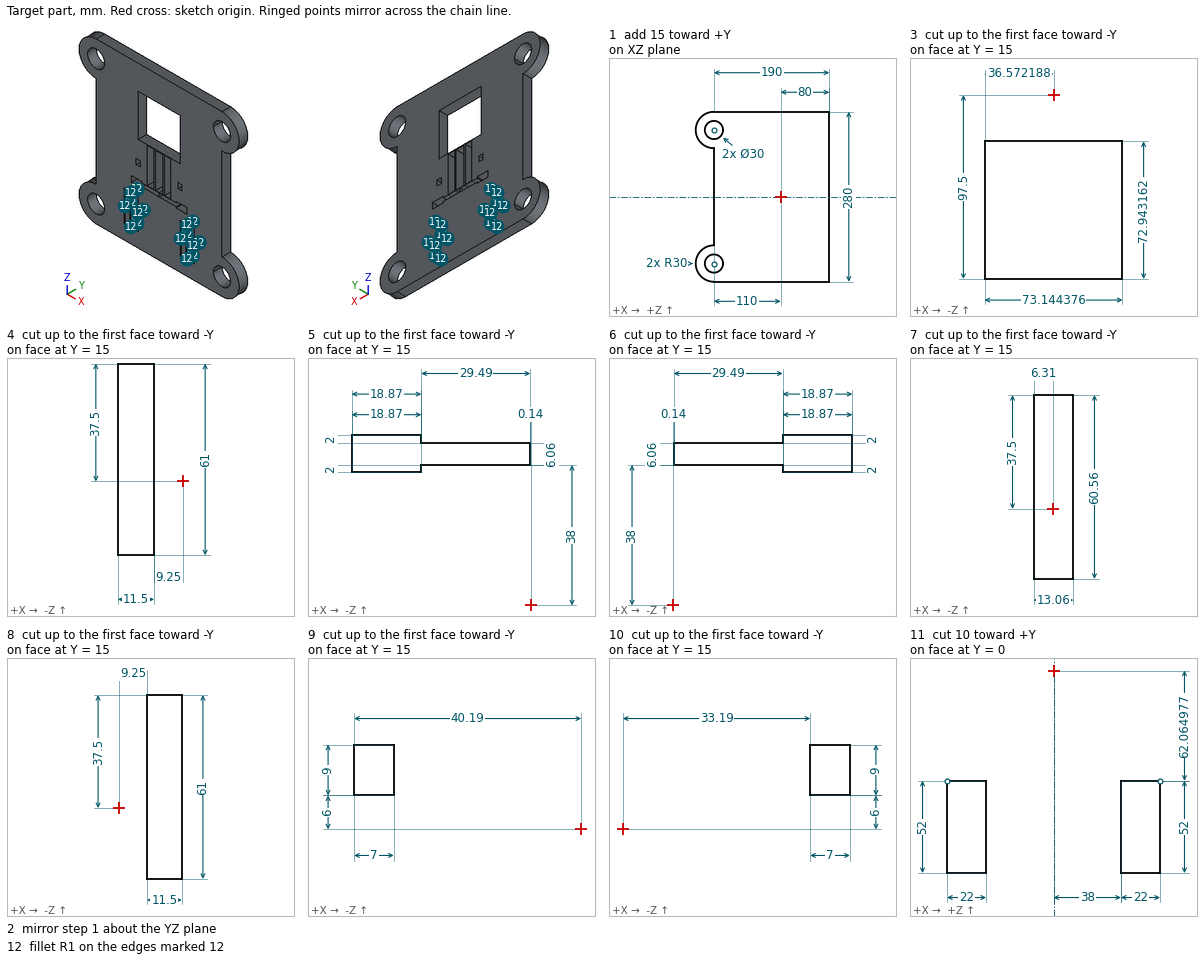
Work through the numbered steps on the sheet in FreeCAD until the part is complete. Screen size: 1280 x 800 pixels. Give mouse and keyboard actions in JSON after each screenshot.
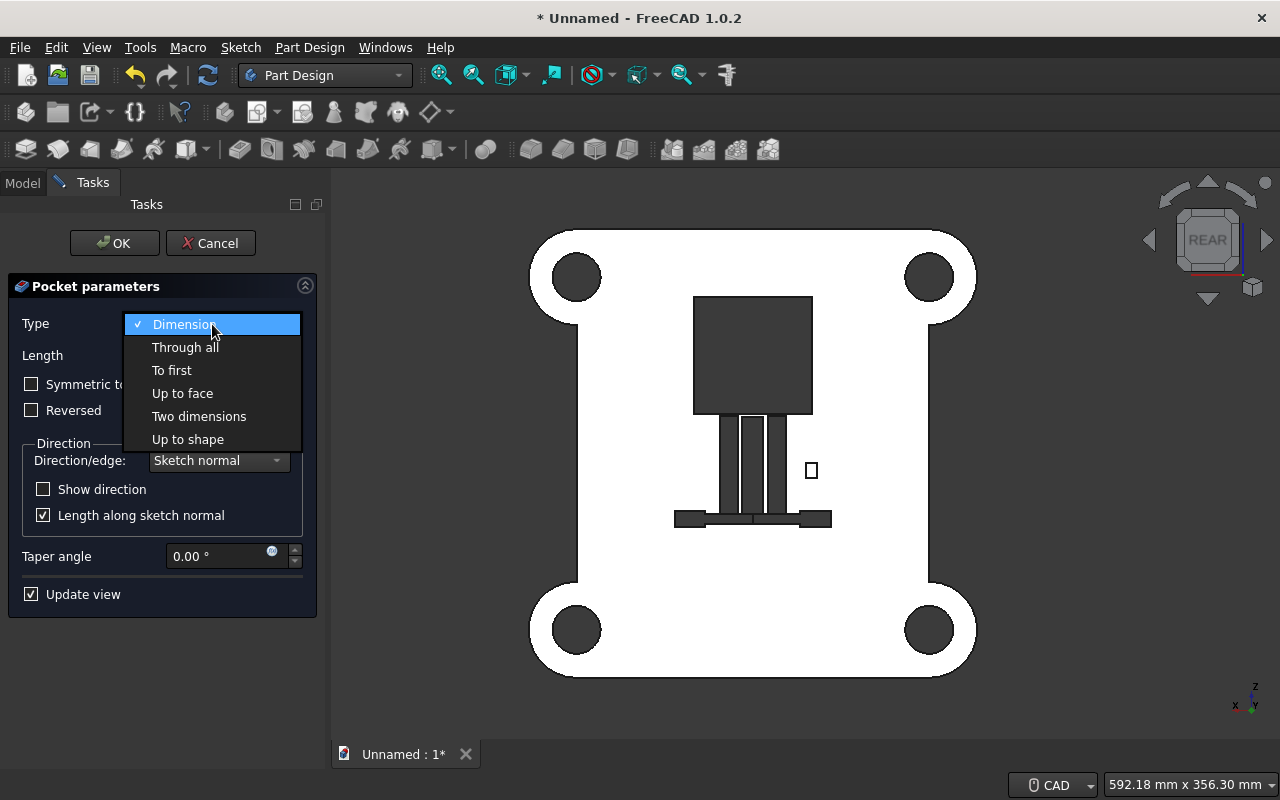
{"action": "left_click", "coordinate": [212, 370]}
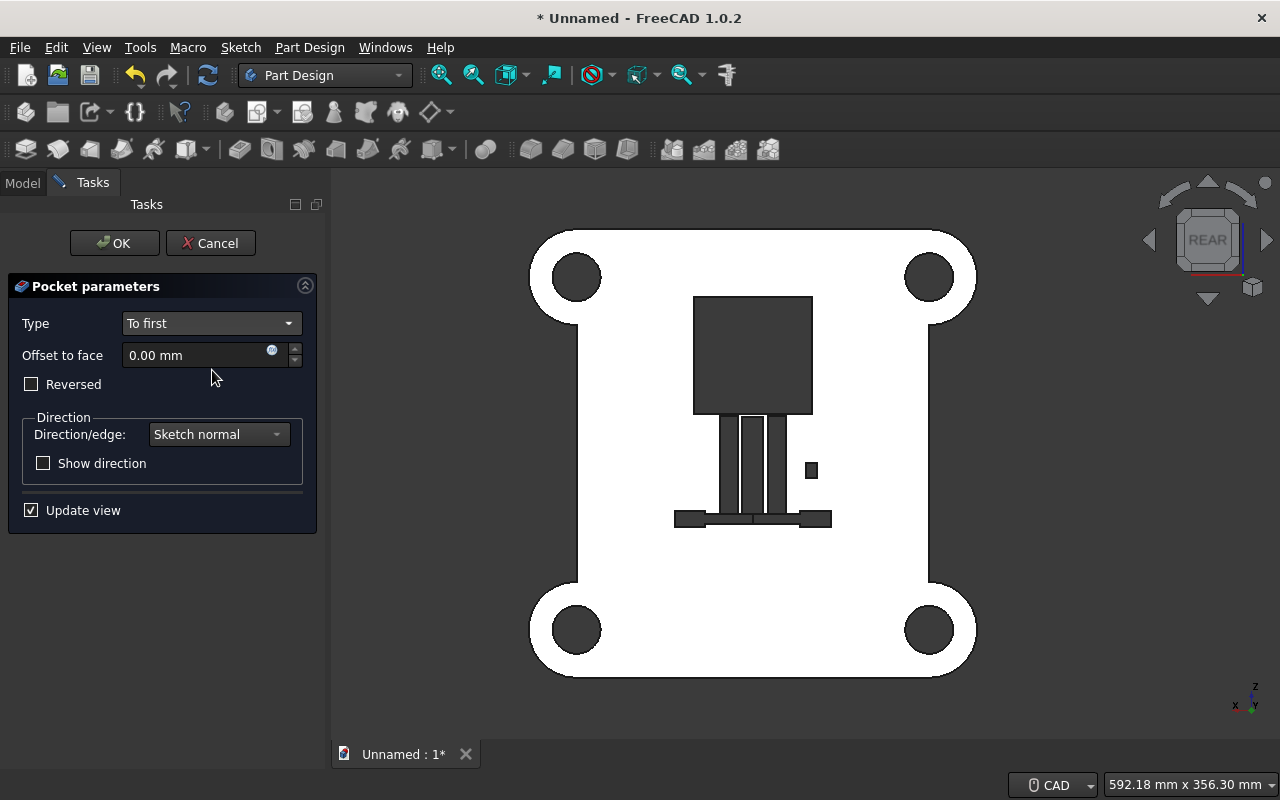
{"action": "left_click", "coordinate": [115, 243]}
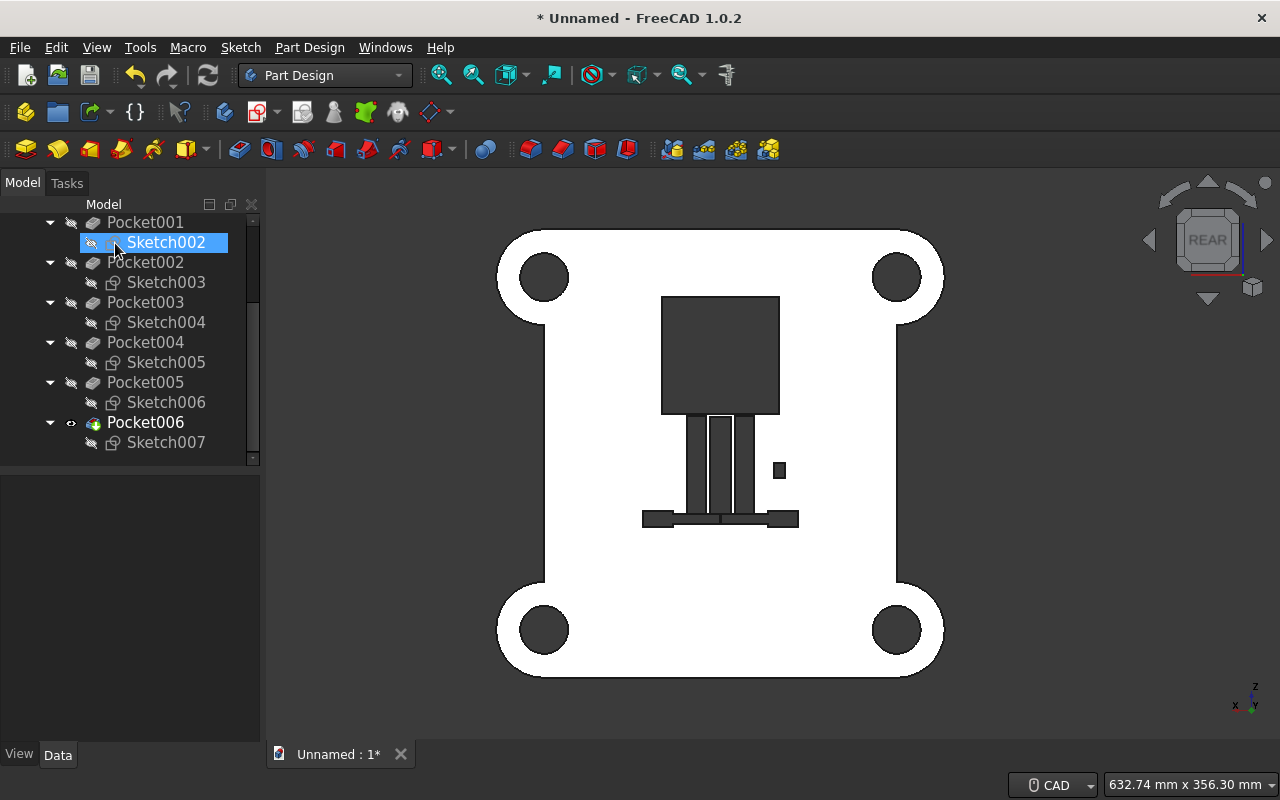
{"action": "left_click", "coordinate": [720, 581]}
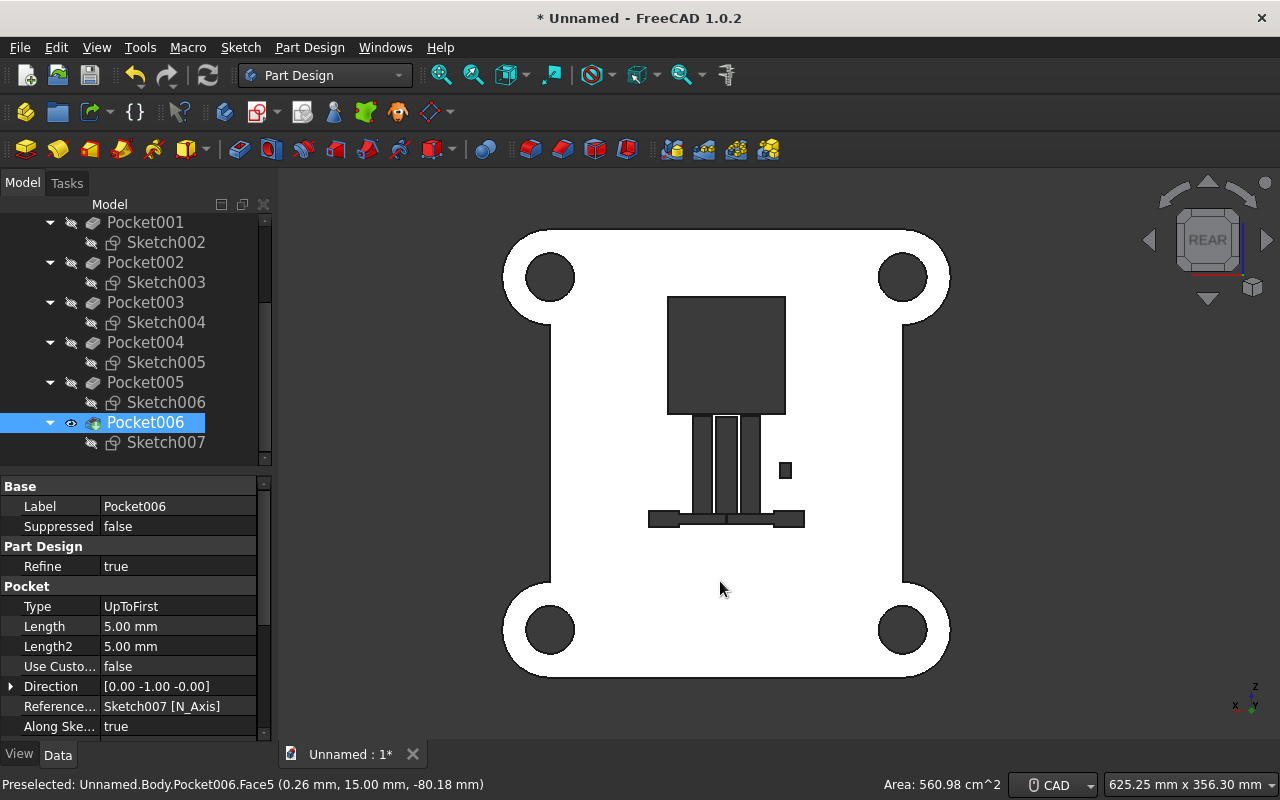
{"action": "left_click", "coordinate": [258, 112]}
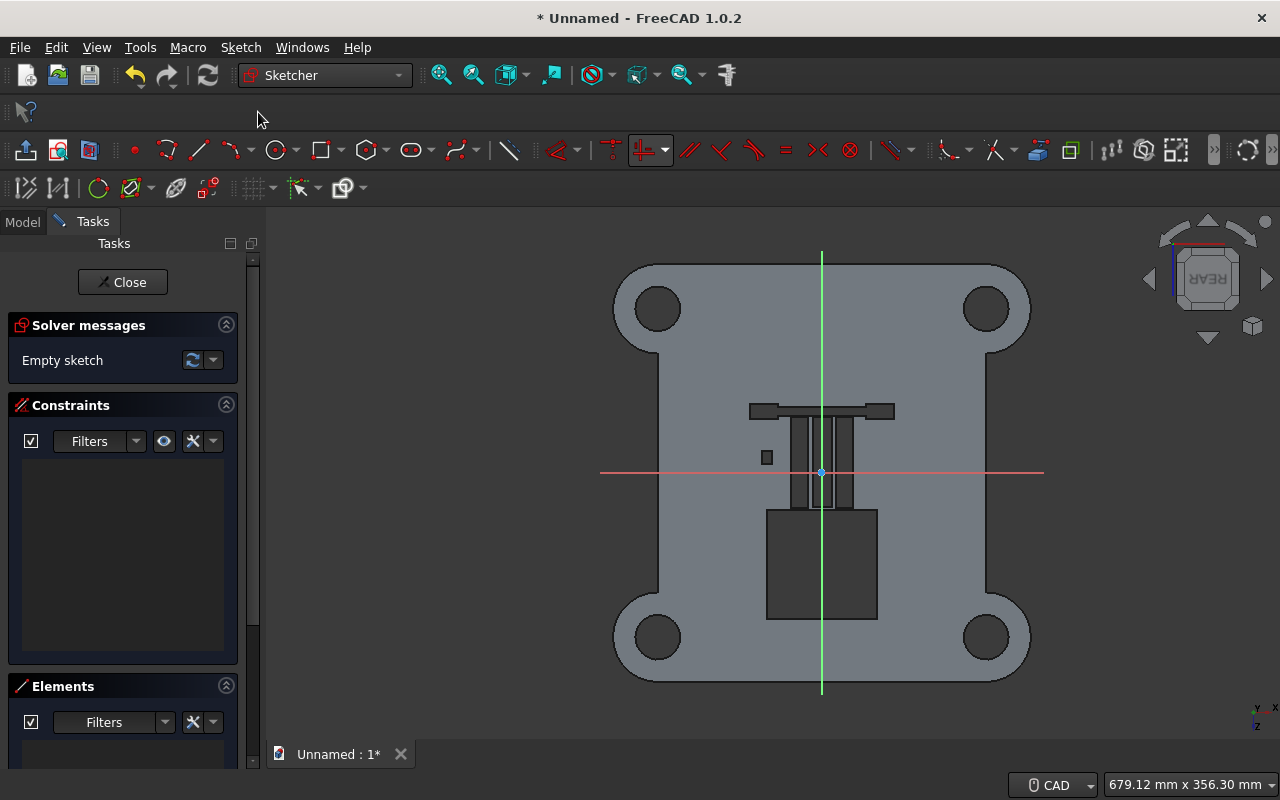
{"action": "scroll", "coordinate": [886, 457], "scroll_direction": "up", "scroll_amount": 15}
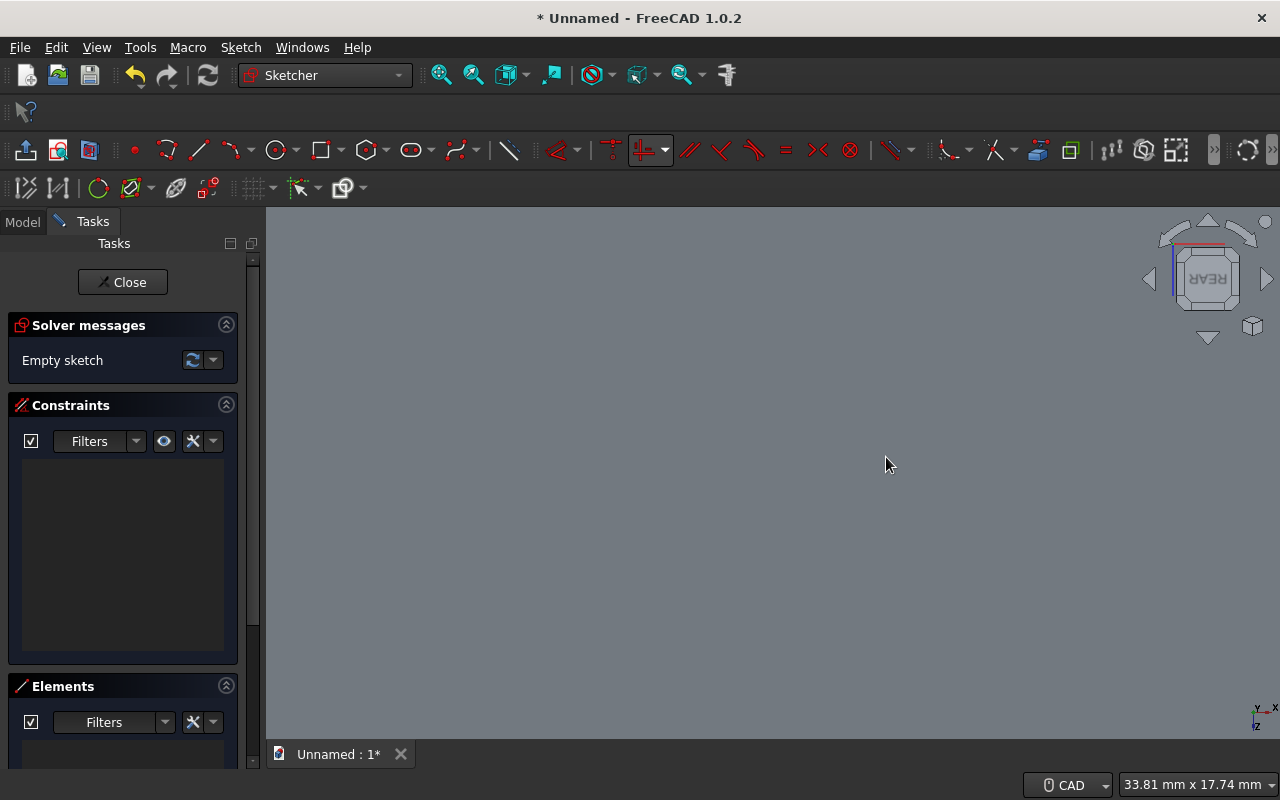
{"action": "key", "text": "g r"}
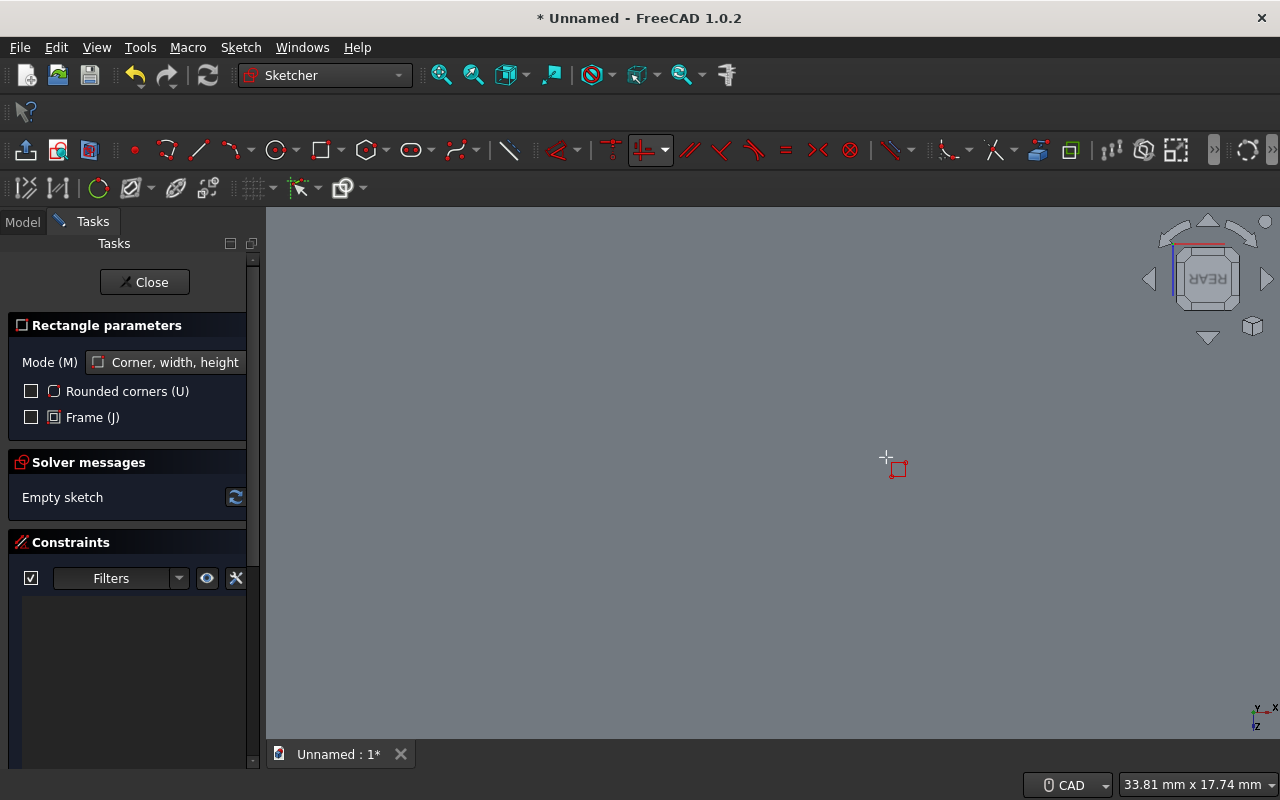
{"action": "left_click", "coordinate": [584, 320]}
{"action": "mouse_move", "coordinate": [794, 589]}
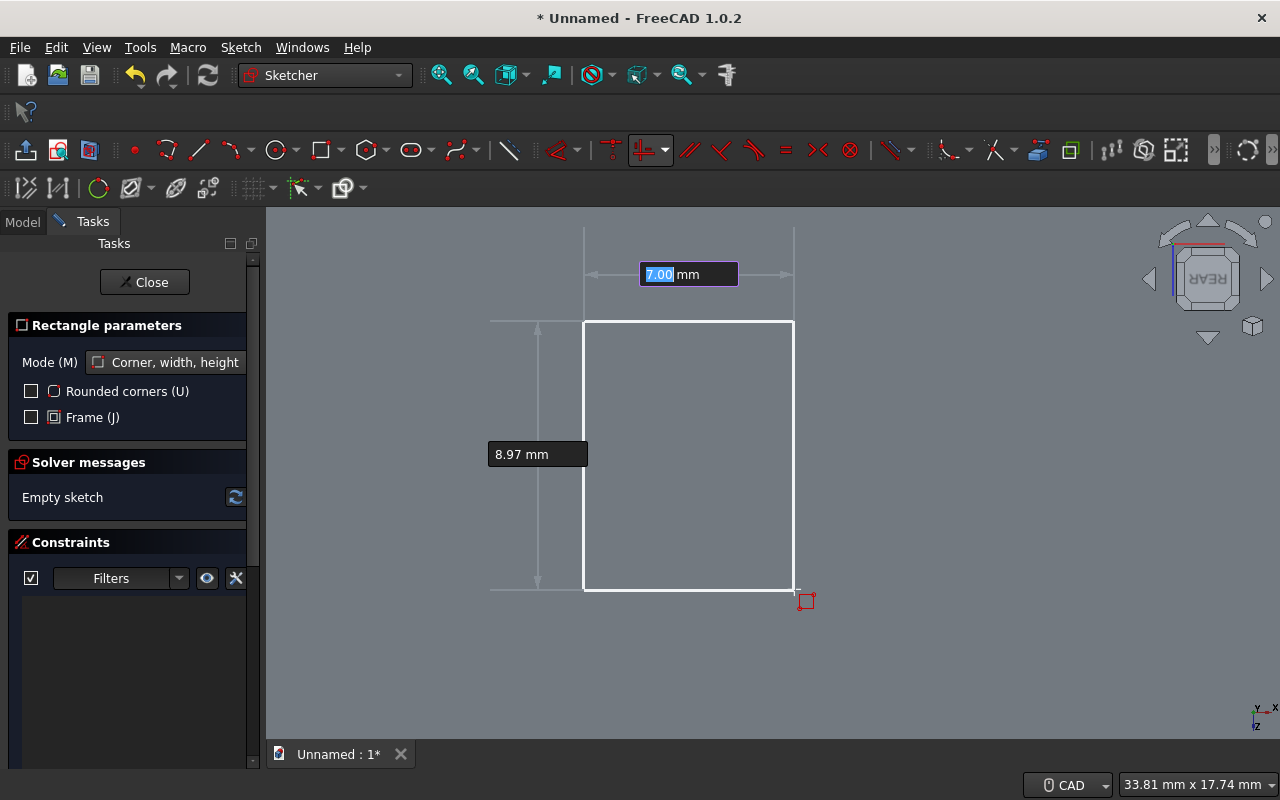
{"action": "type", "text": "7"}
{"action": "key", "text": "Tab"}
{"action": "type", "text": "9"}
{"action": "key", "text": "Return"}
{"action": "key", "text": "Escape"}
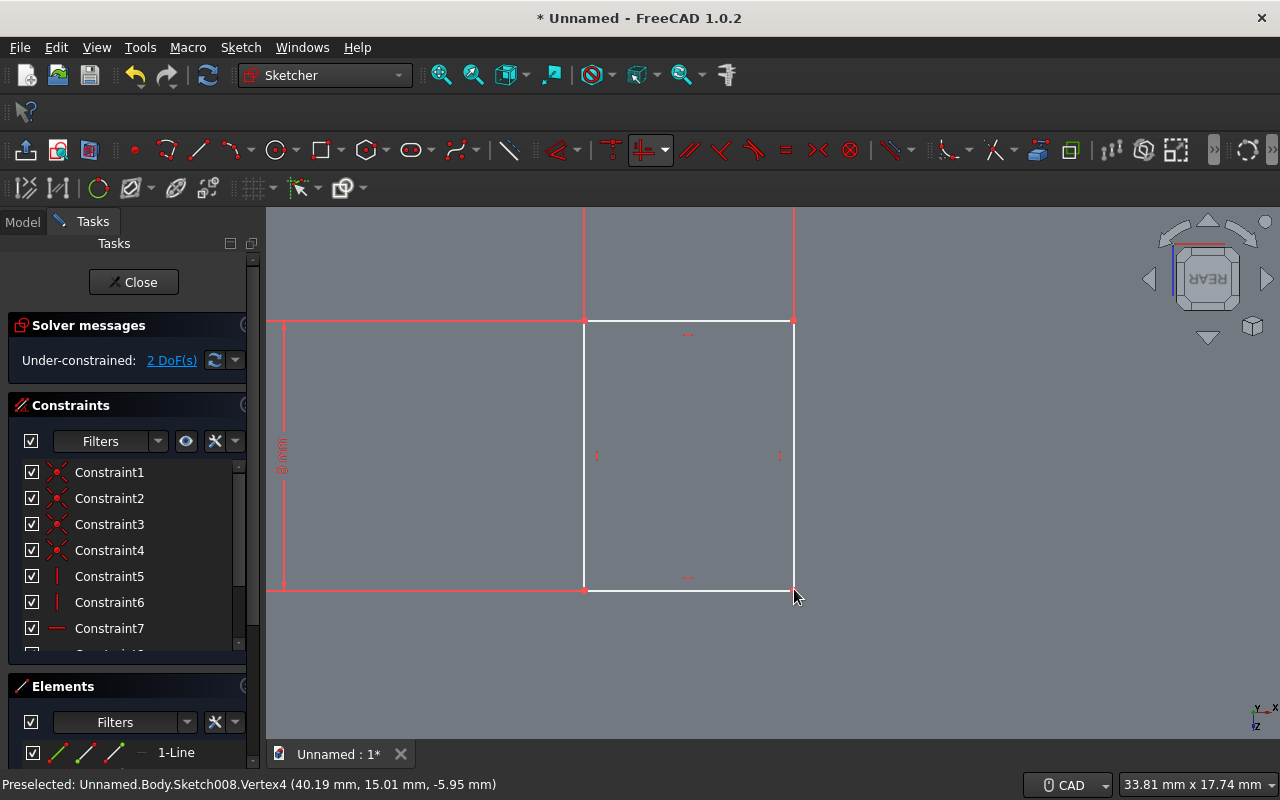
{"action": "left_click", "coordinate": [556, 150]}